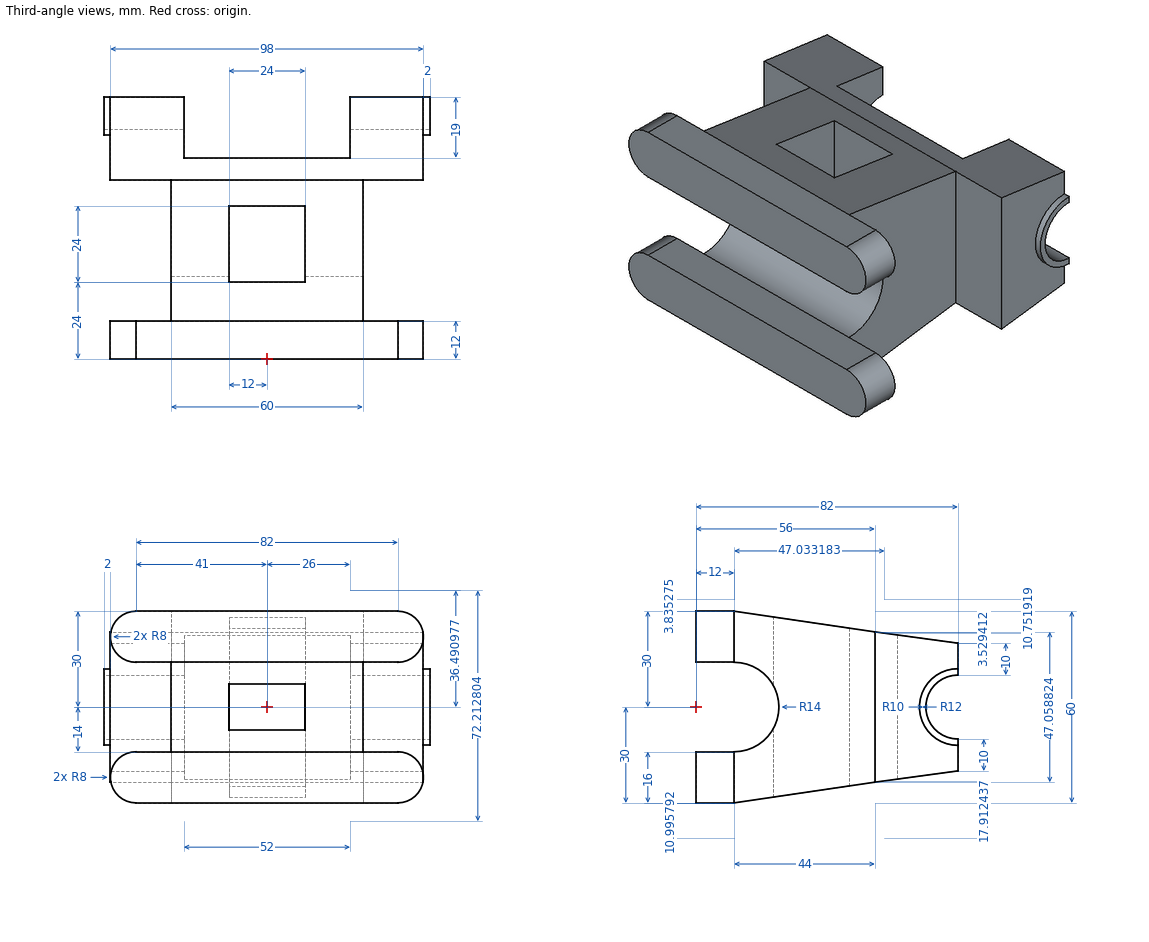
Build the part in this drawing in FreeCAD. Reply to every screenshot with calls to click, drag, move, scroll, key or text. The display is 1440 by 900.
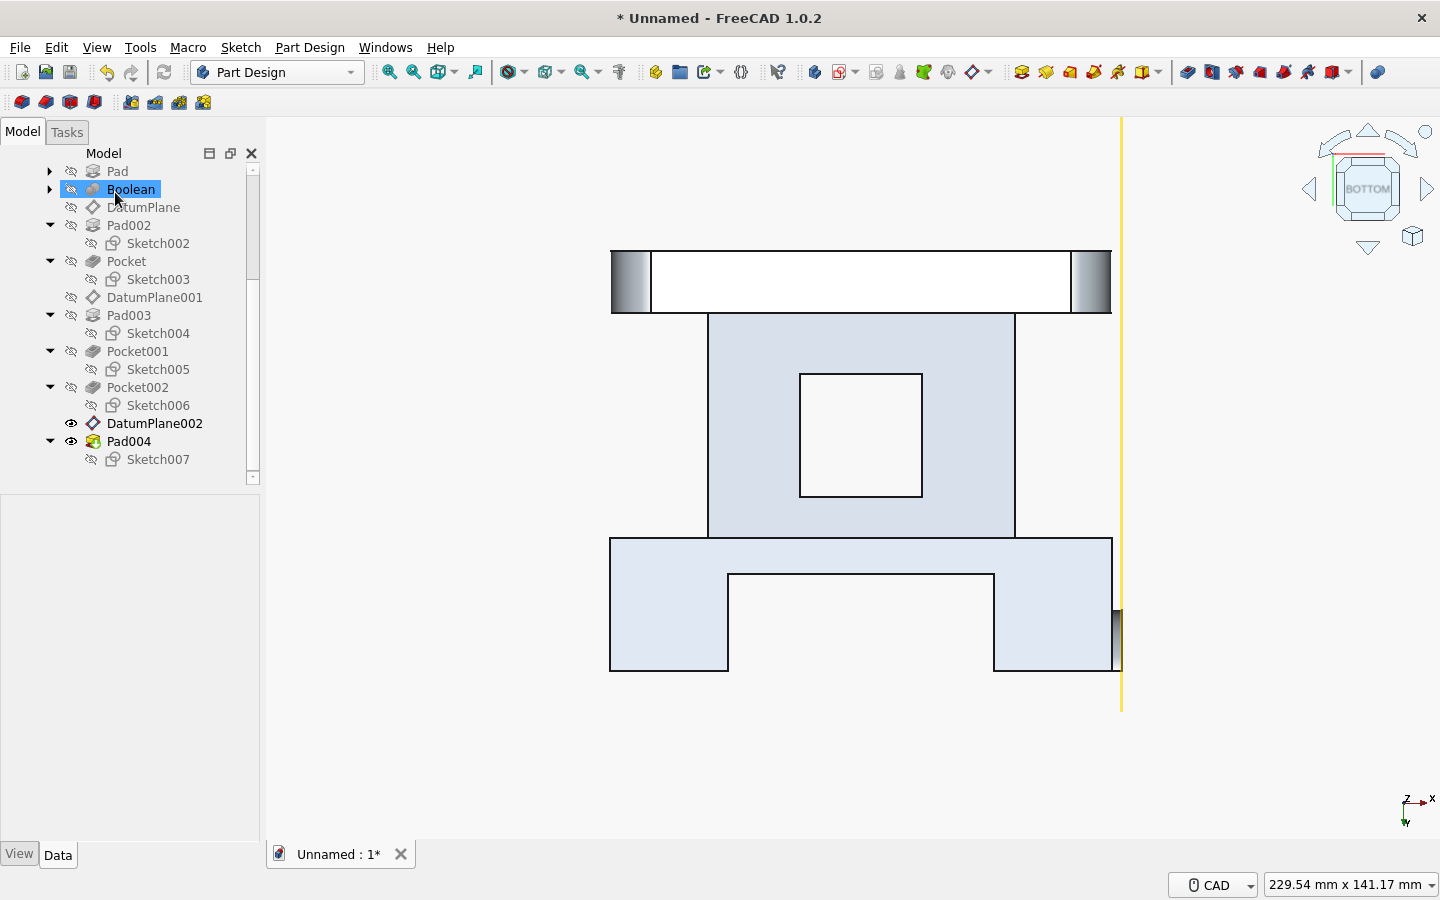
click(116, 423)
key(space)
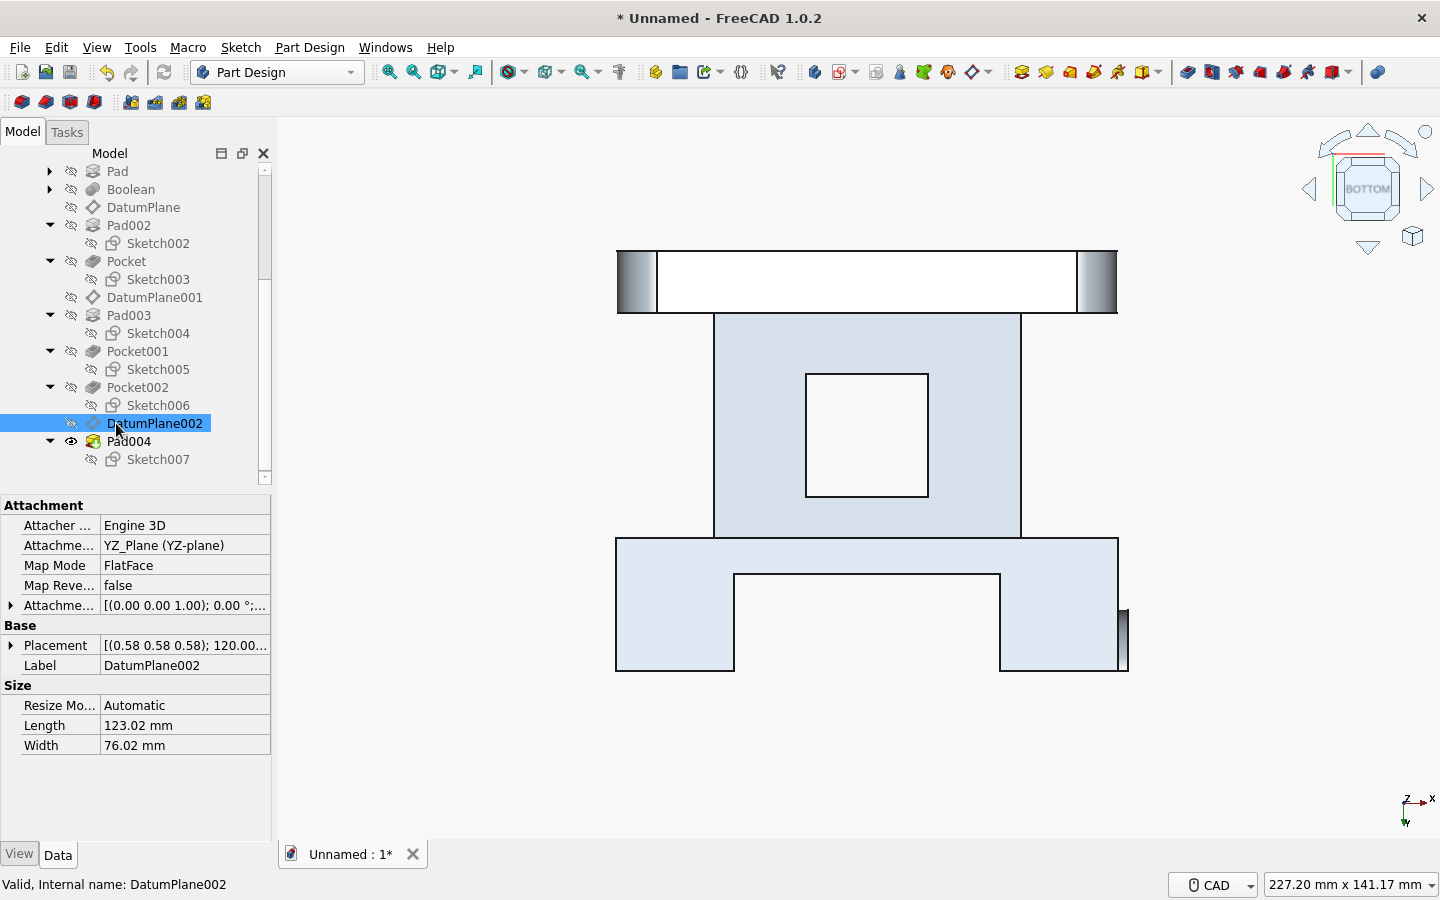
key(6)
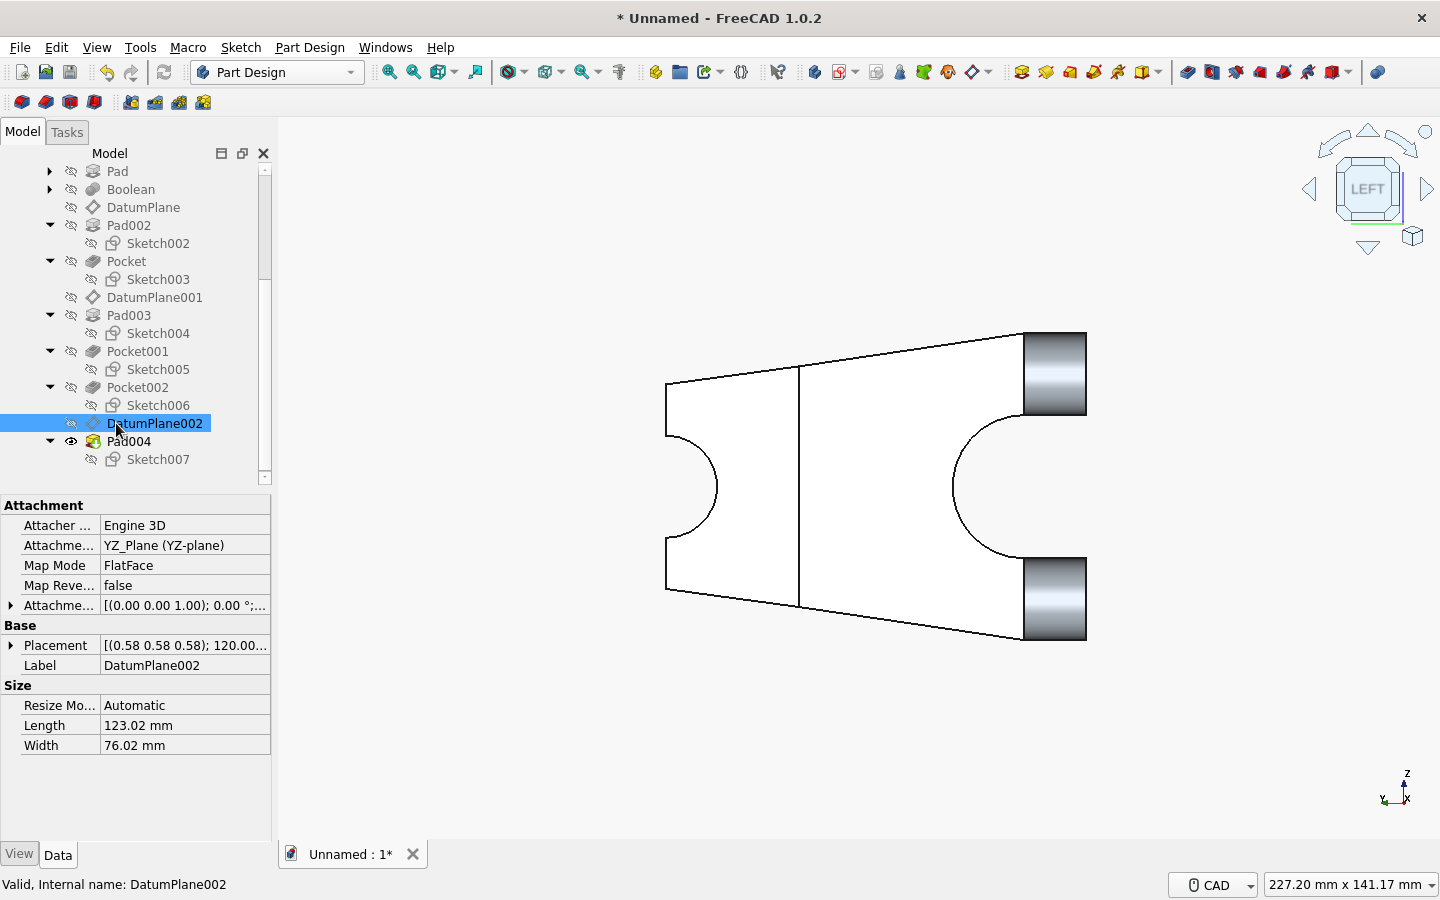
click(390, 72)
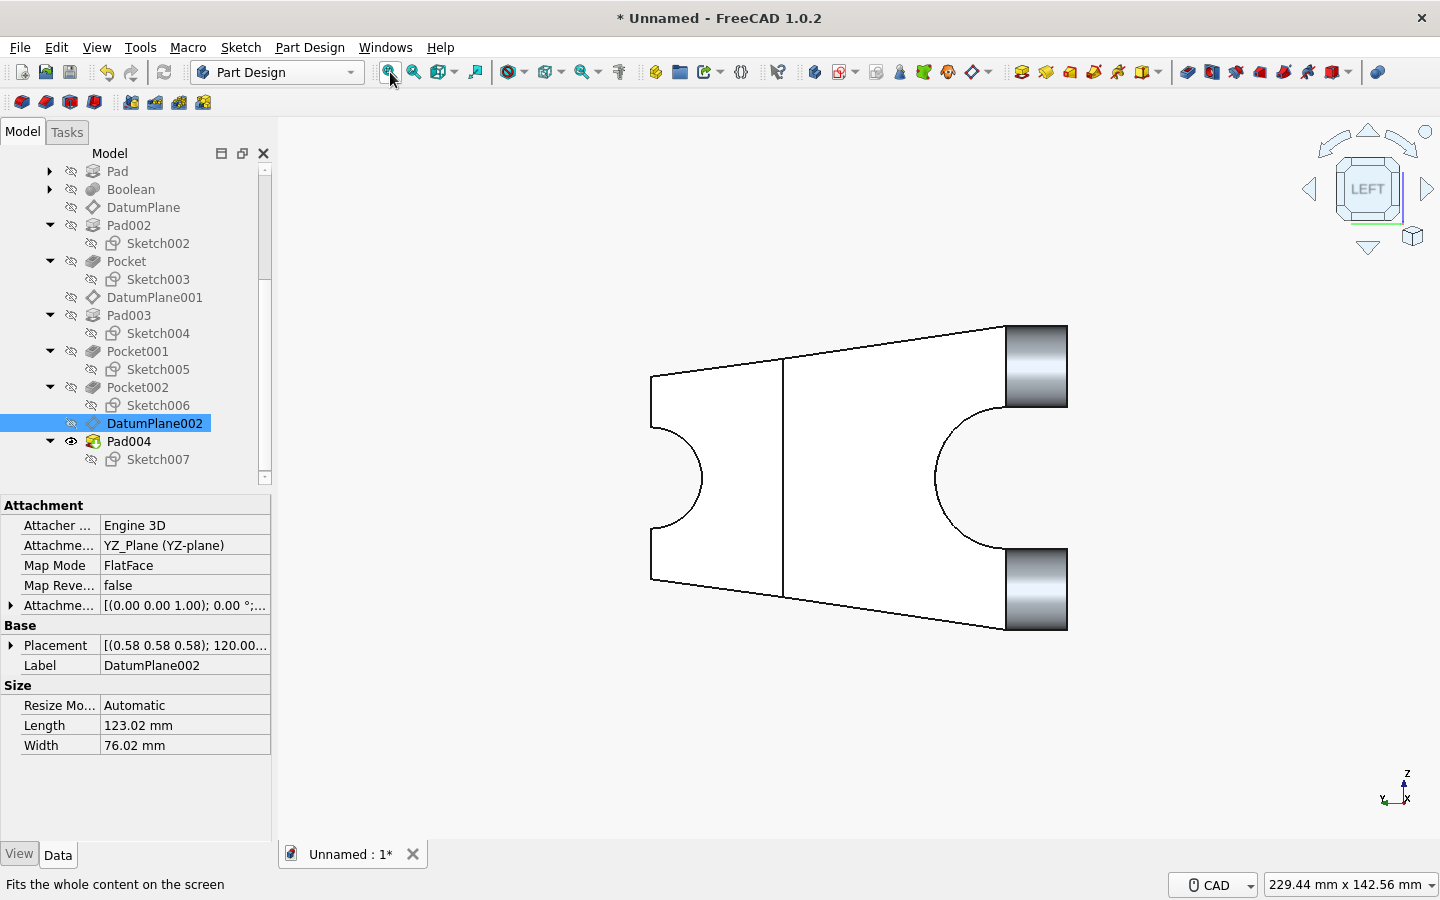
click(736, 409)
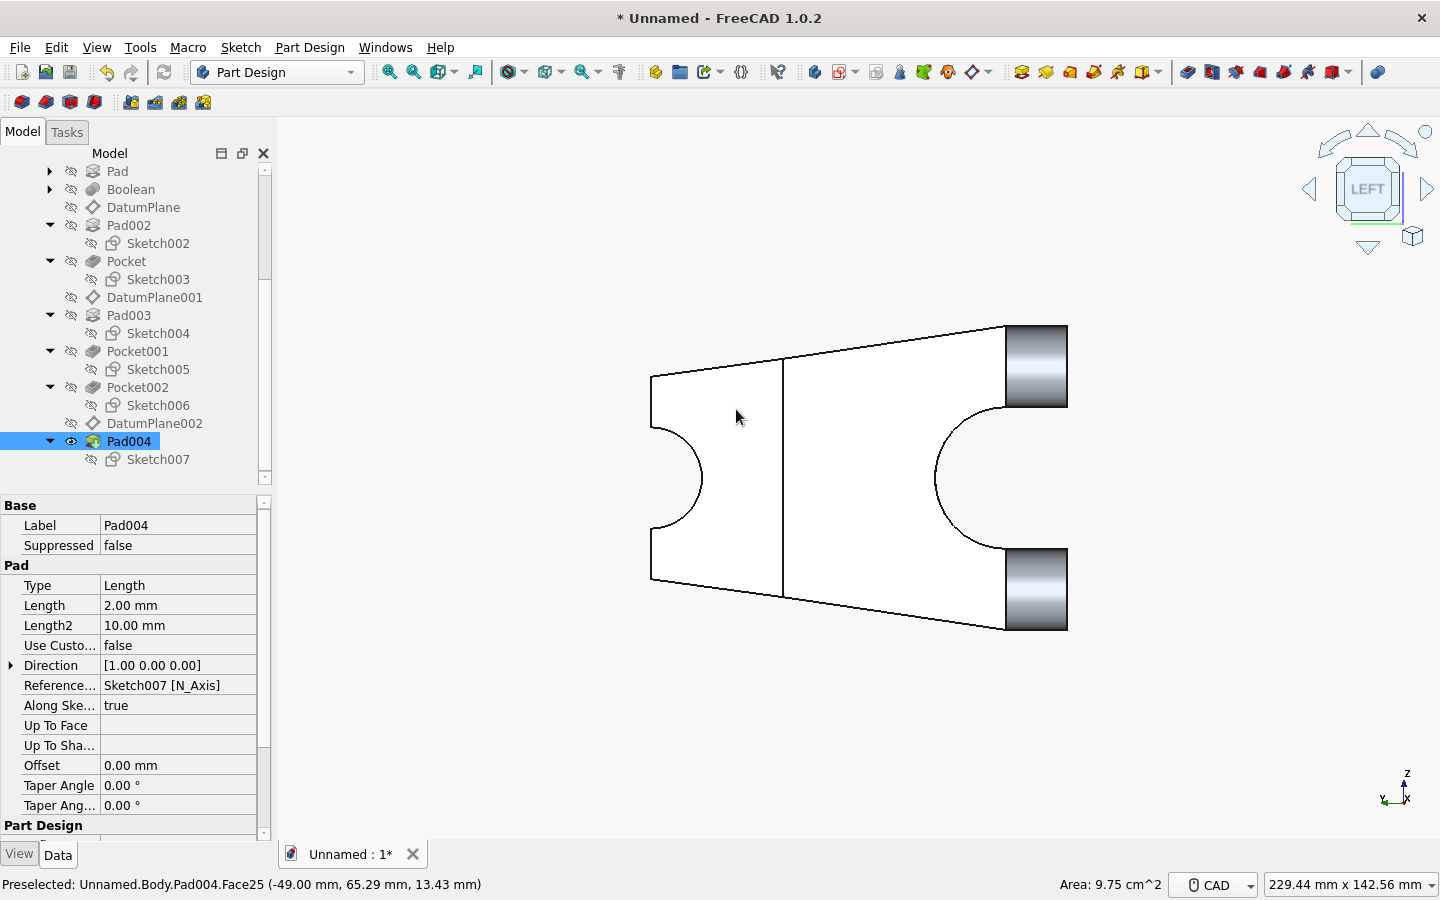
click(840, 72)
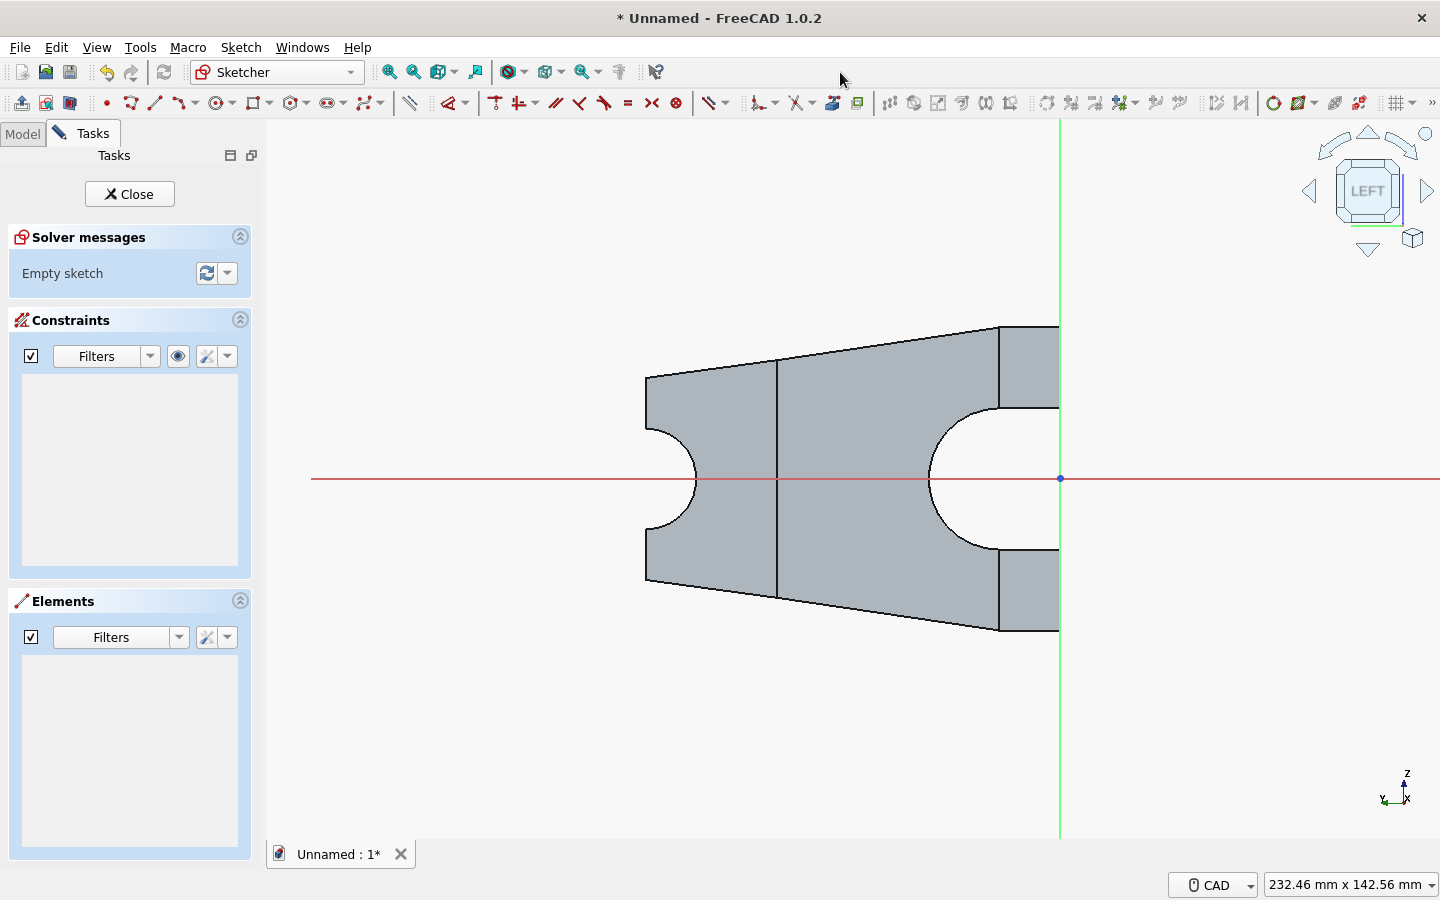
scroll(641, 479, up, 7)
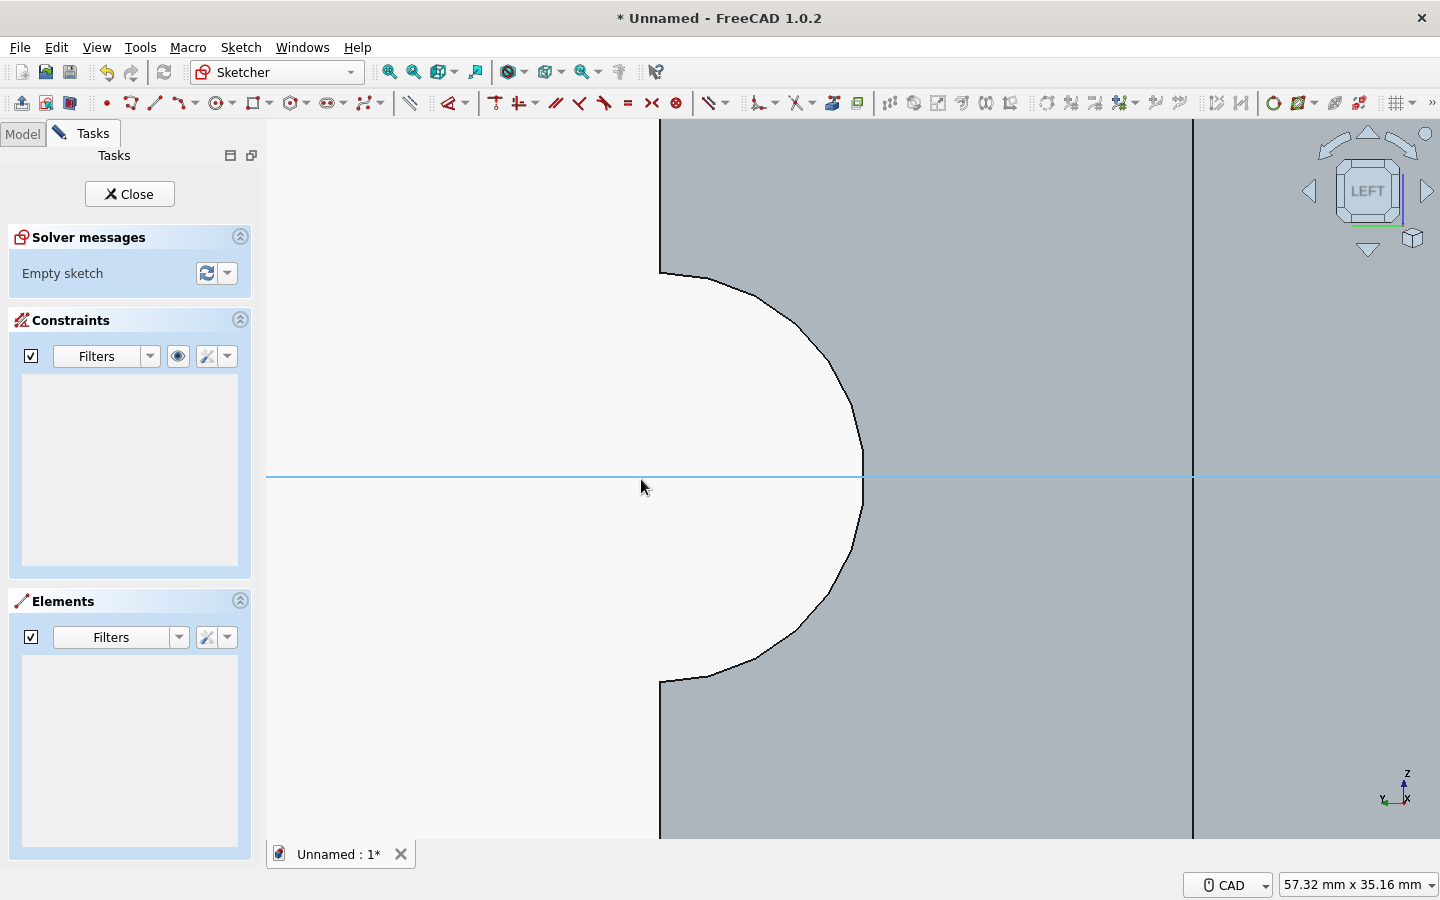
click(156, 104)